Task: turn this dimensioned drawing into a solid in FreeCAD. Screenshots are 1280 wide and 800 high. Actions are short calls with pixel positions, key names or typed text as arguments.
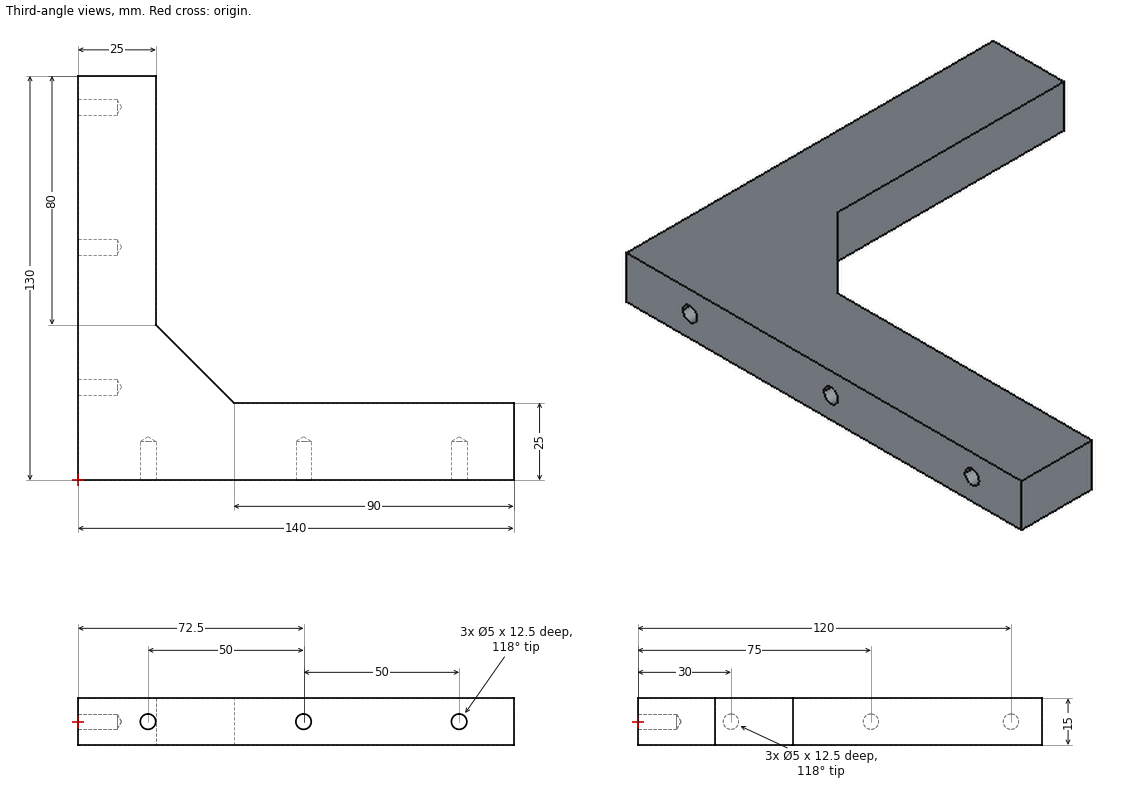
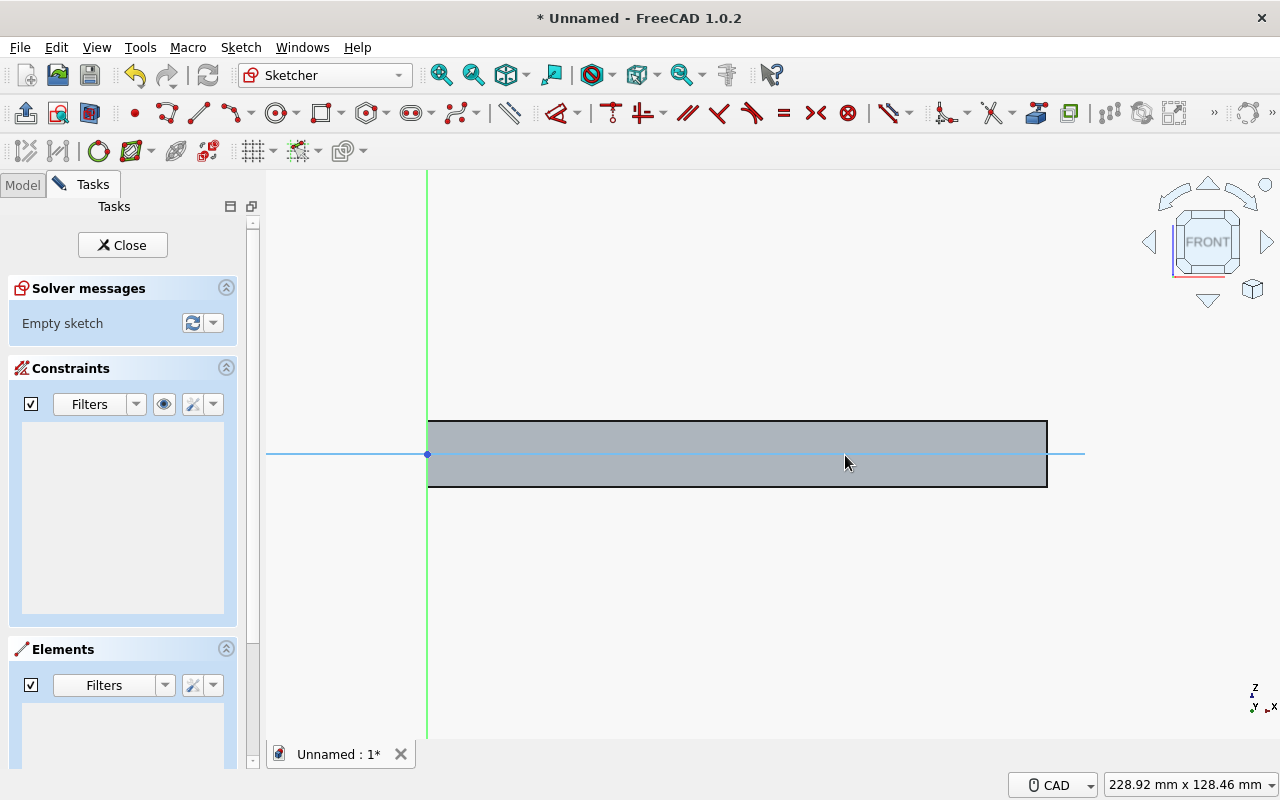
click(276, 114)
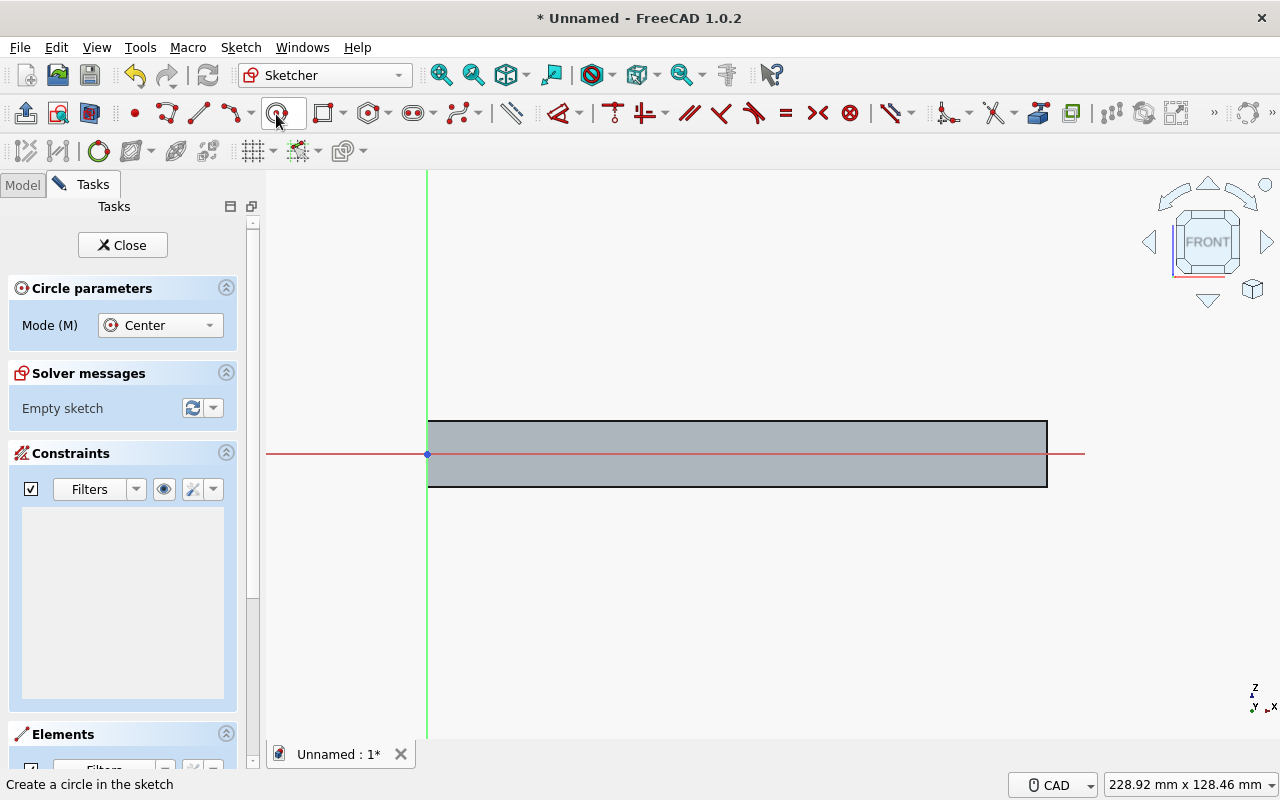
scroll(970, 454, up, 4)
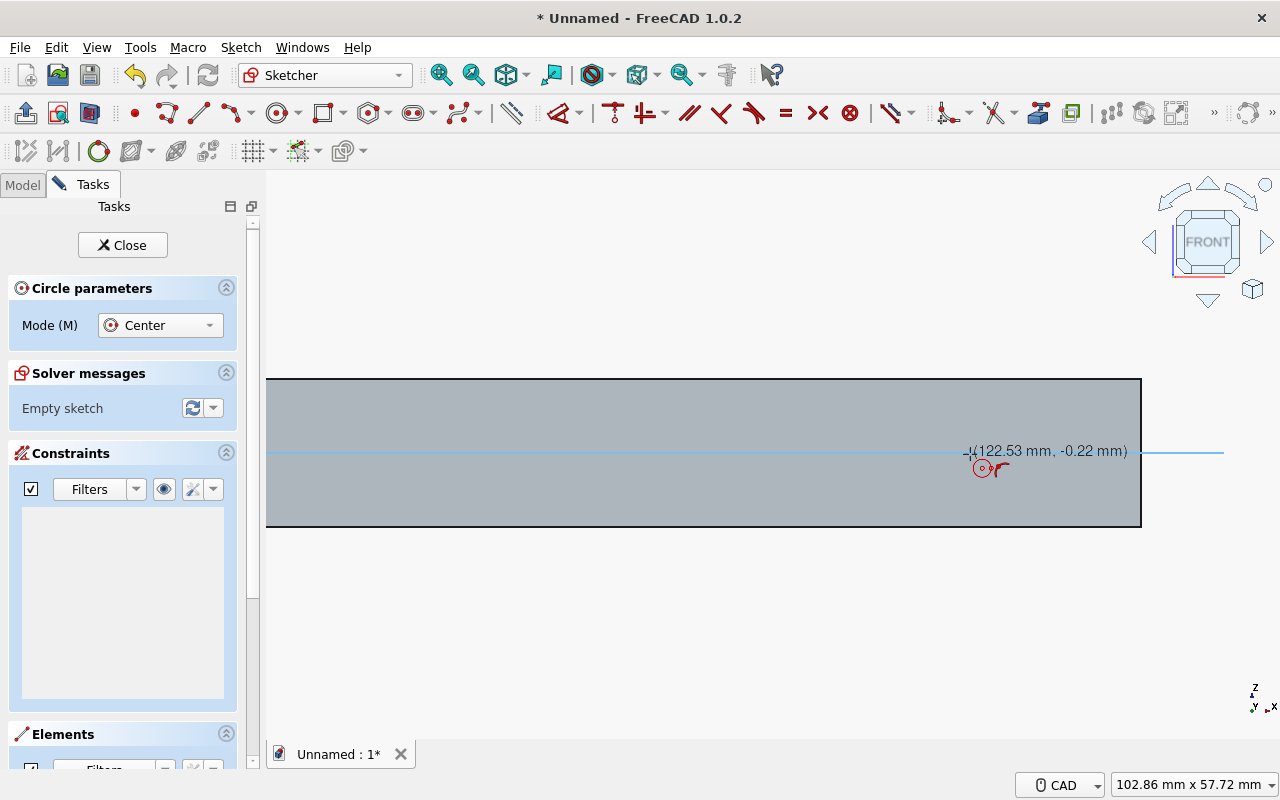
click(969, 453)
click(986, 436)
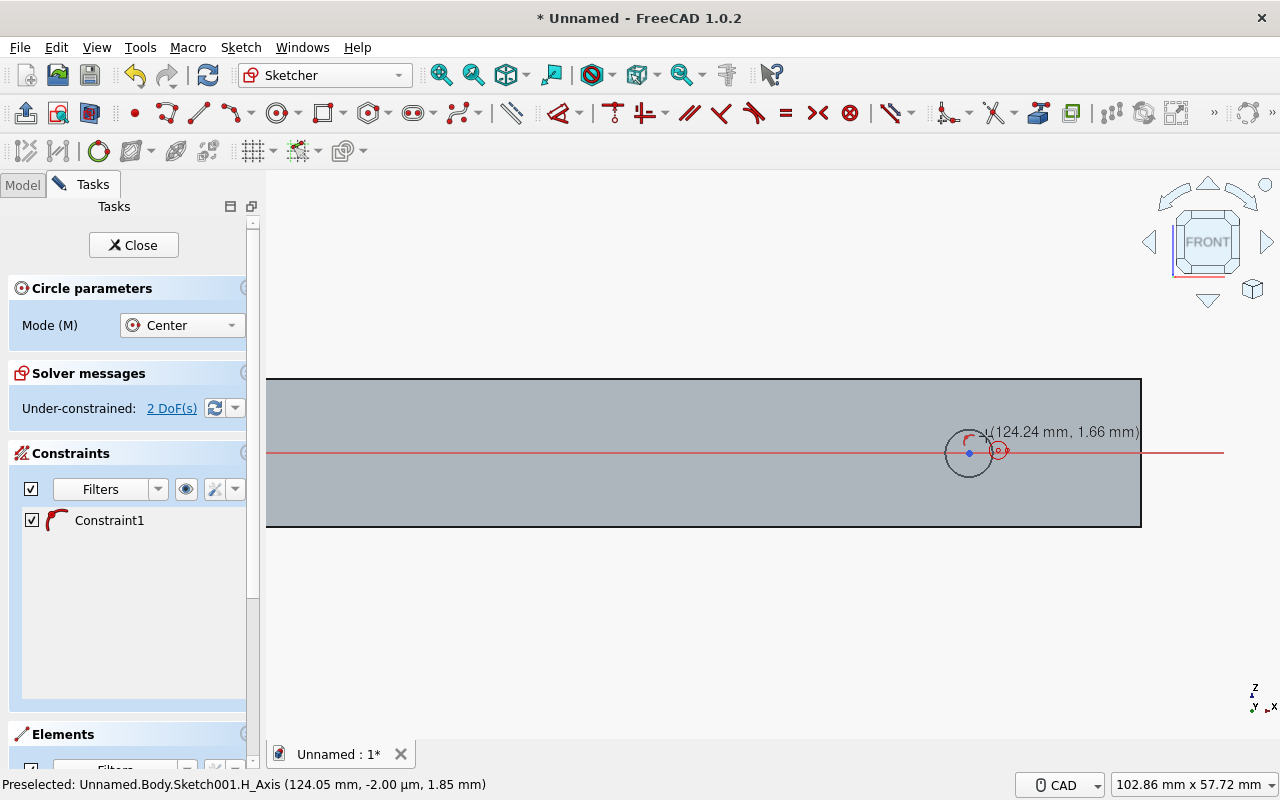
click(476, 453)
click(493, 436)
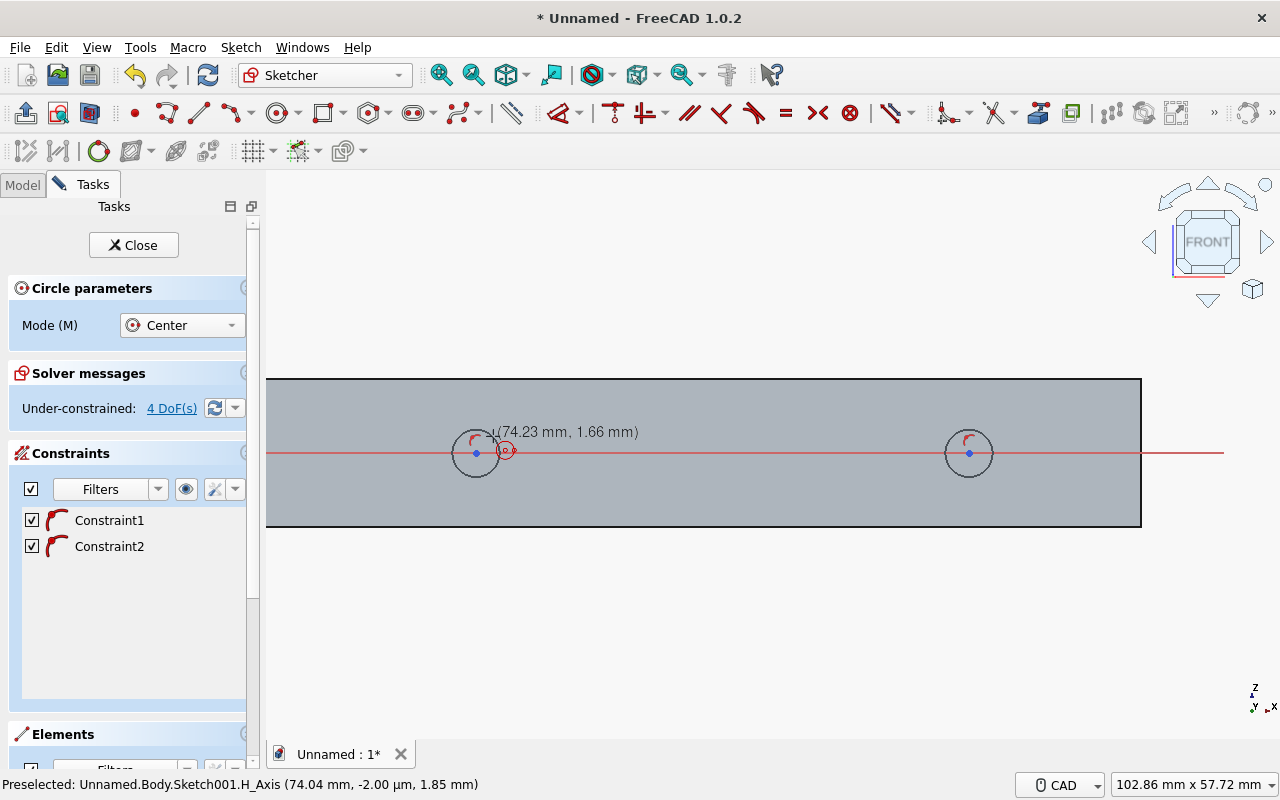
scroll(971, 455, down, 4)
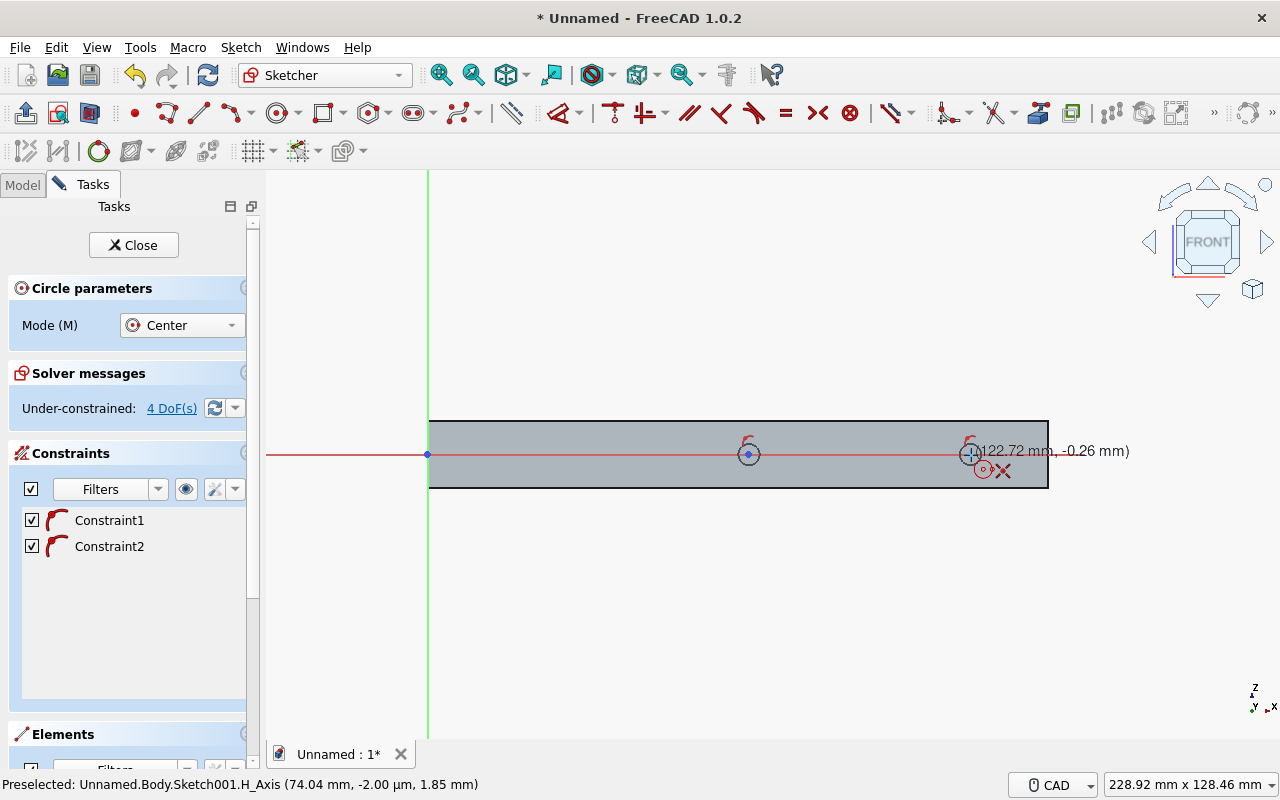
scroll(527, 455, up, 4)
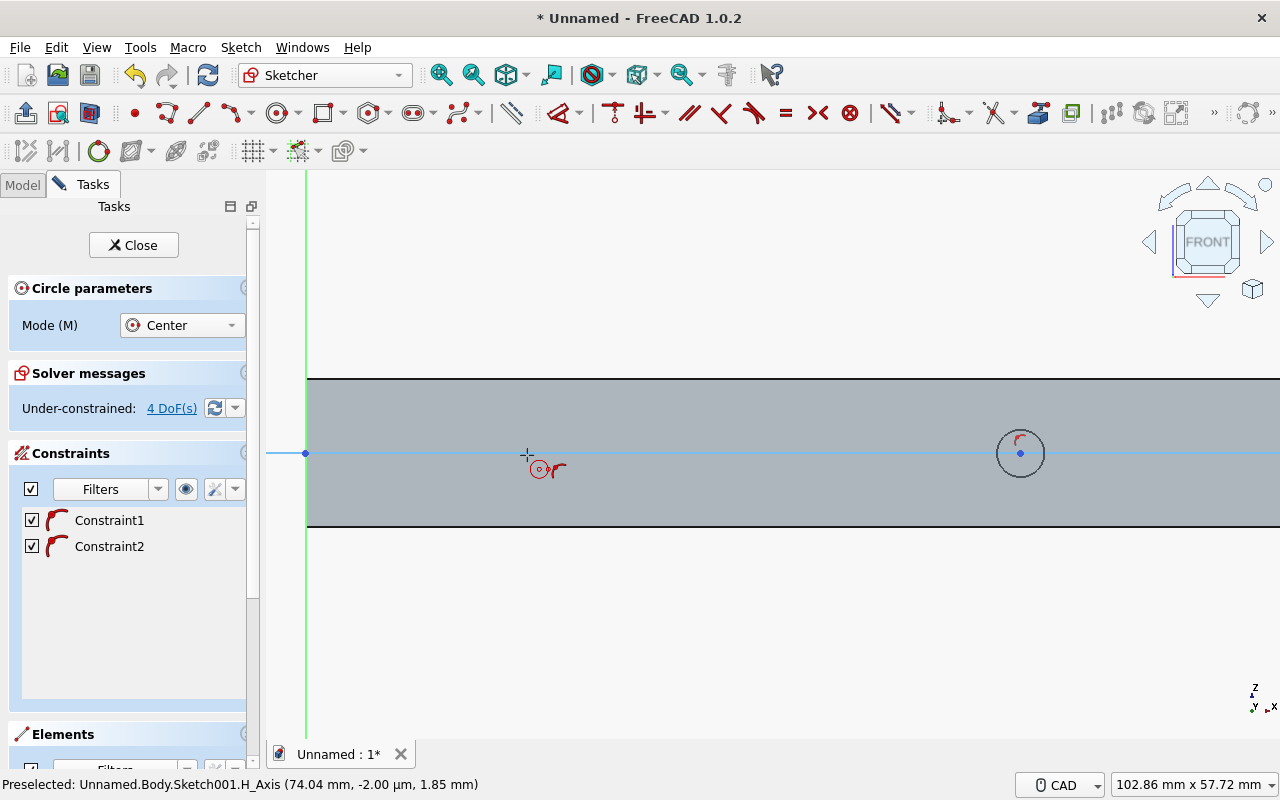
click(528, 453)
click(545, 436)
key(Escape)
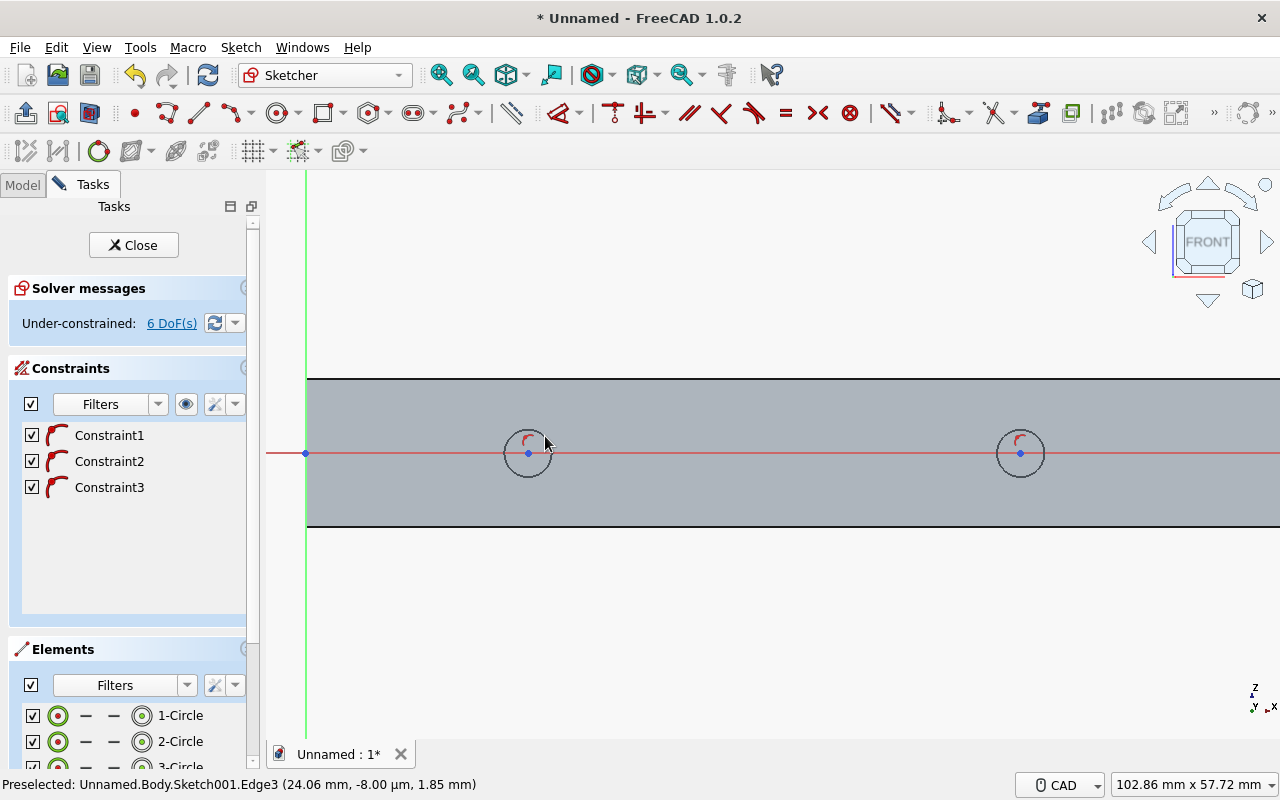
scroll(527, 455, down, 4)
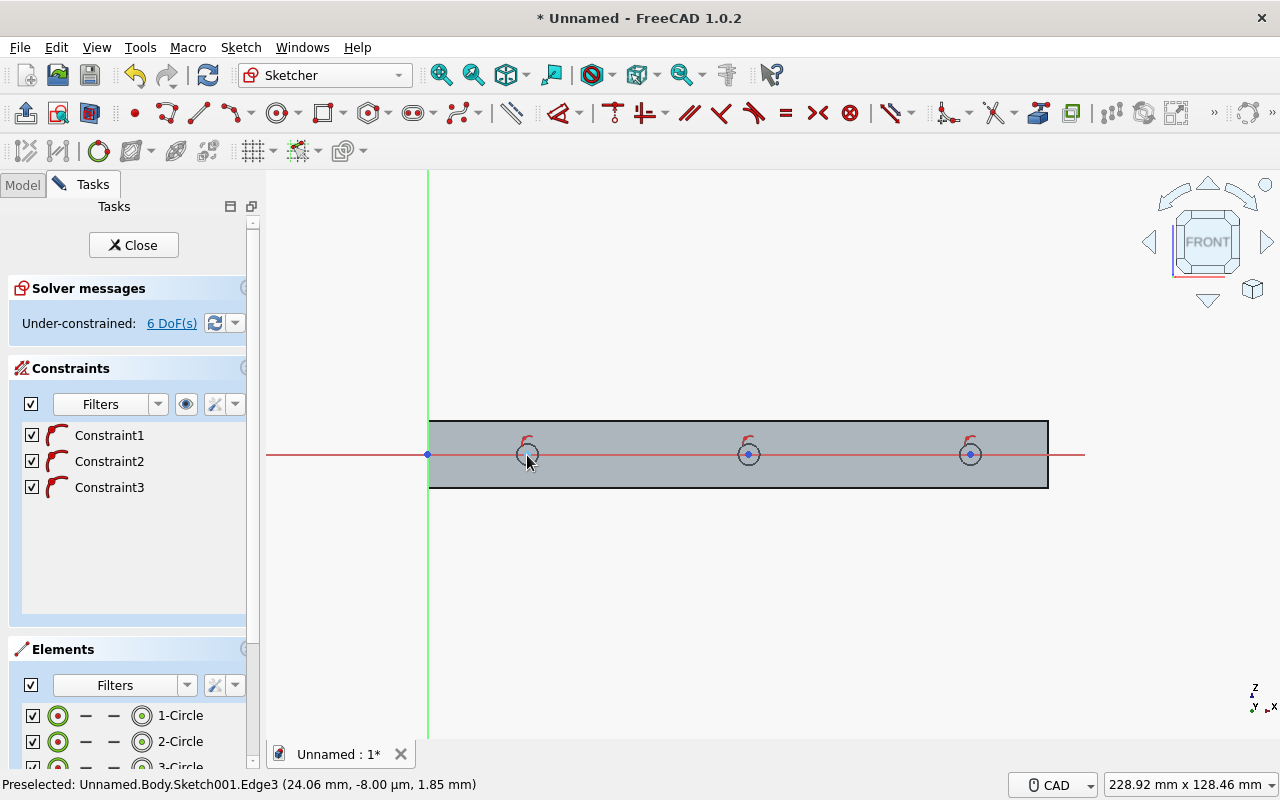
scroll(978, 447, up, 4)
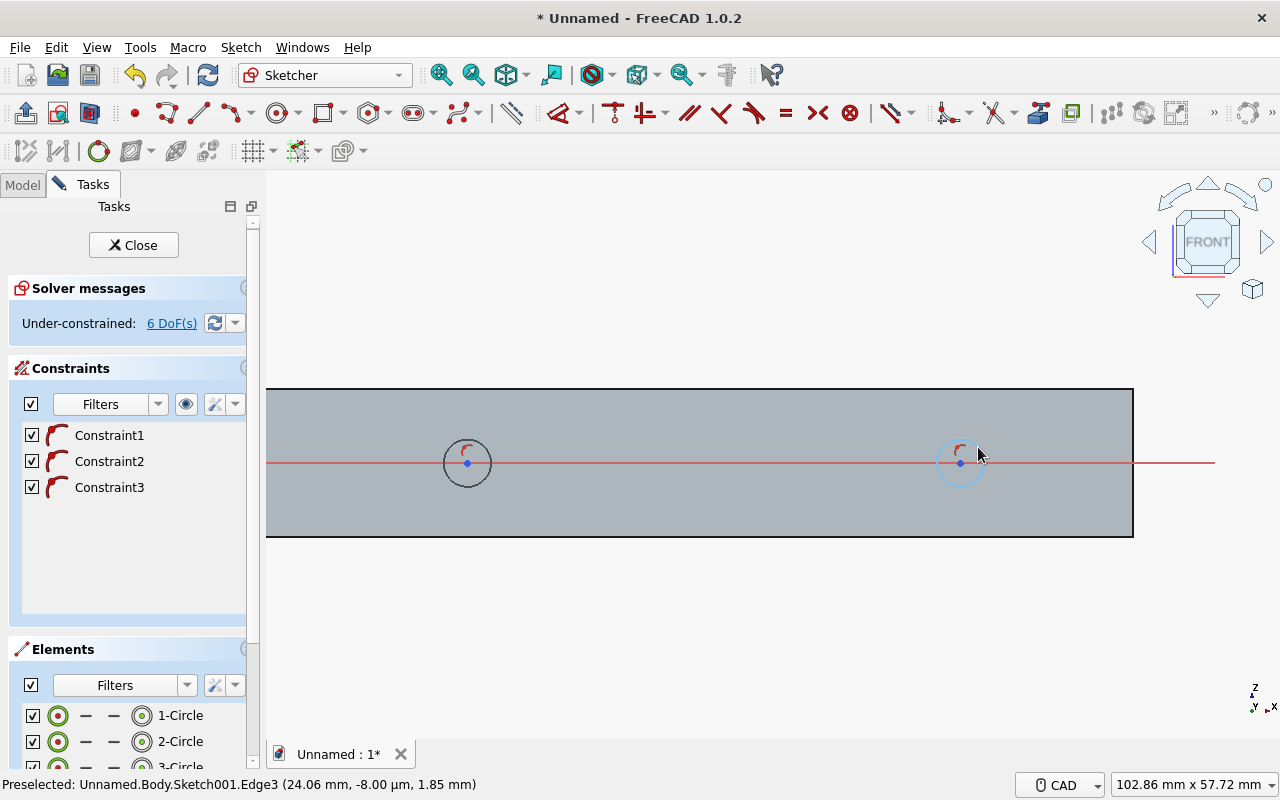
click(977, 446)